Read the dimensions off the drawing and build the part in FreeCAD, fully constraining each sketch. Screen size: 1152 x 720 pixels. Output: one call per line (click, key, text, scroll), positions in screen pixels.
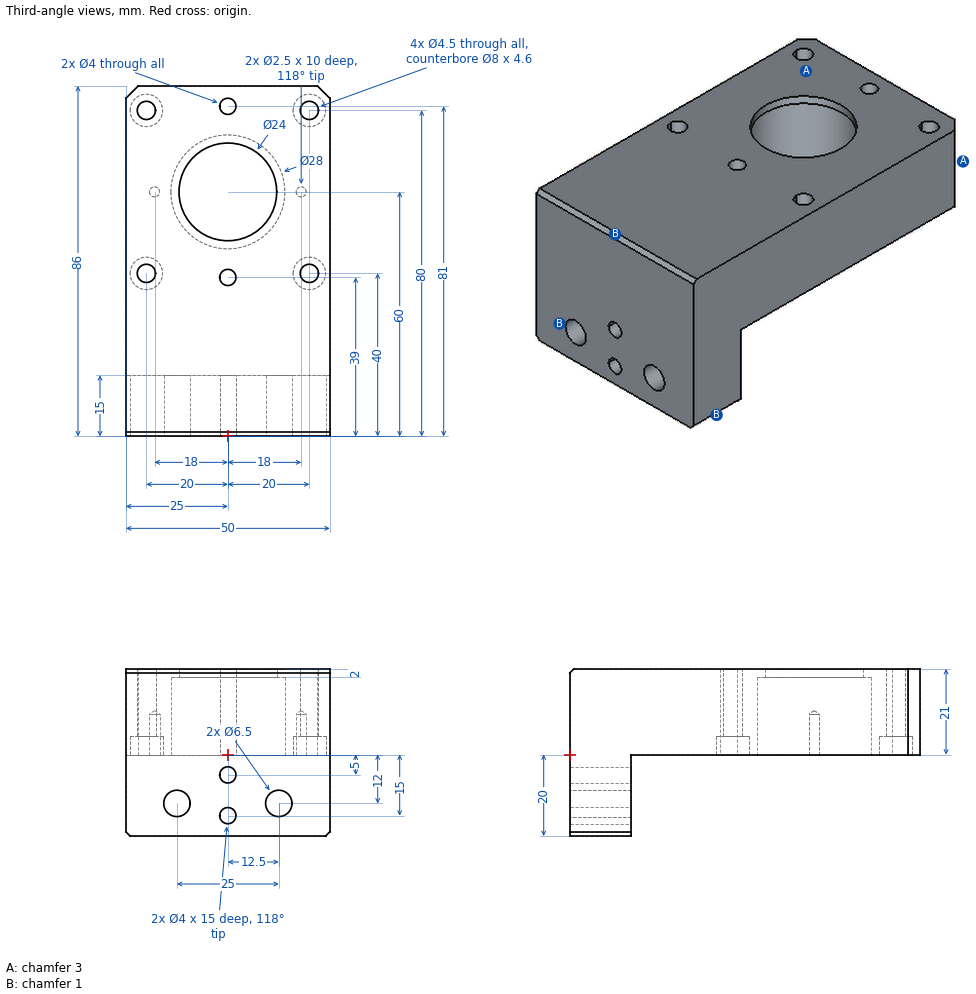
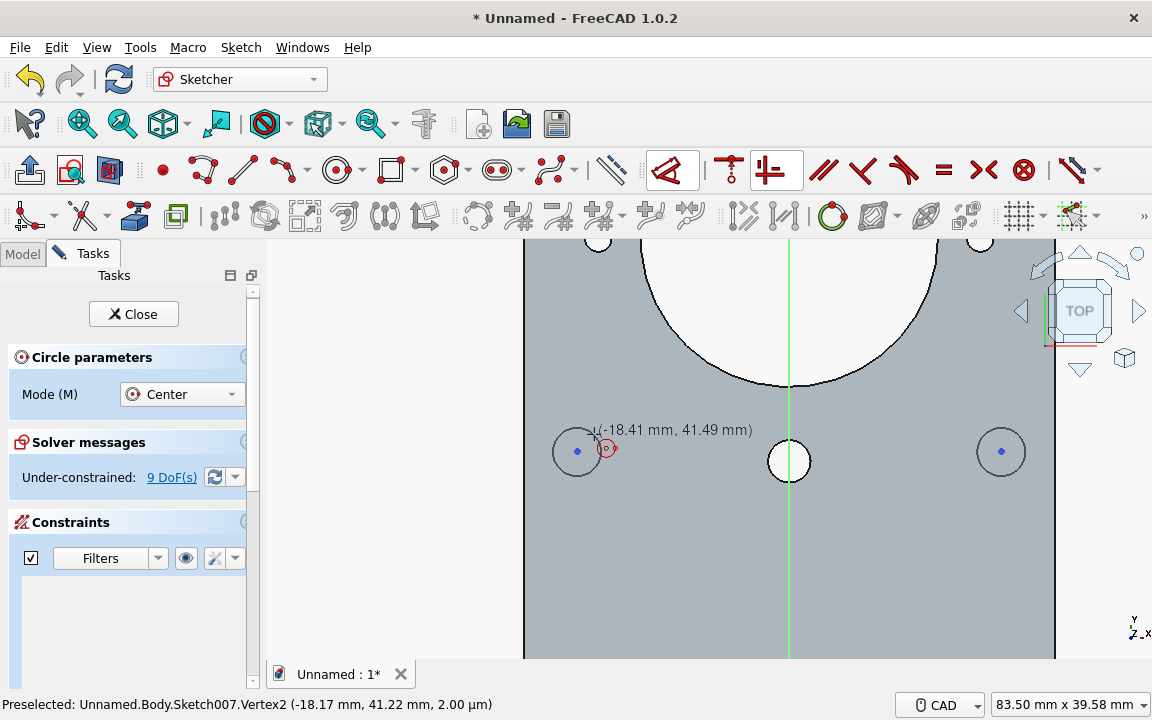
scroll(576, 453, down, 6)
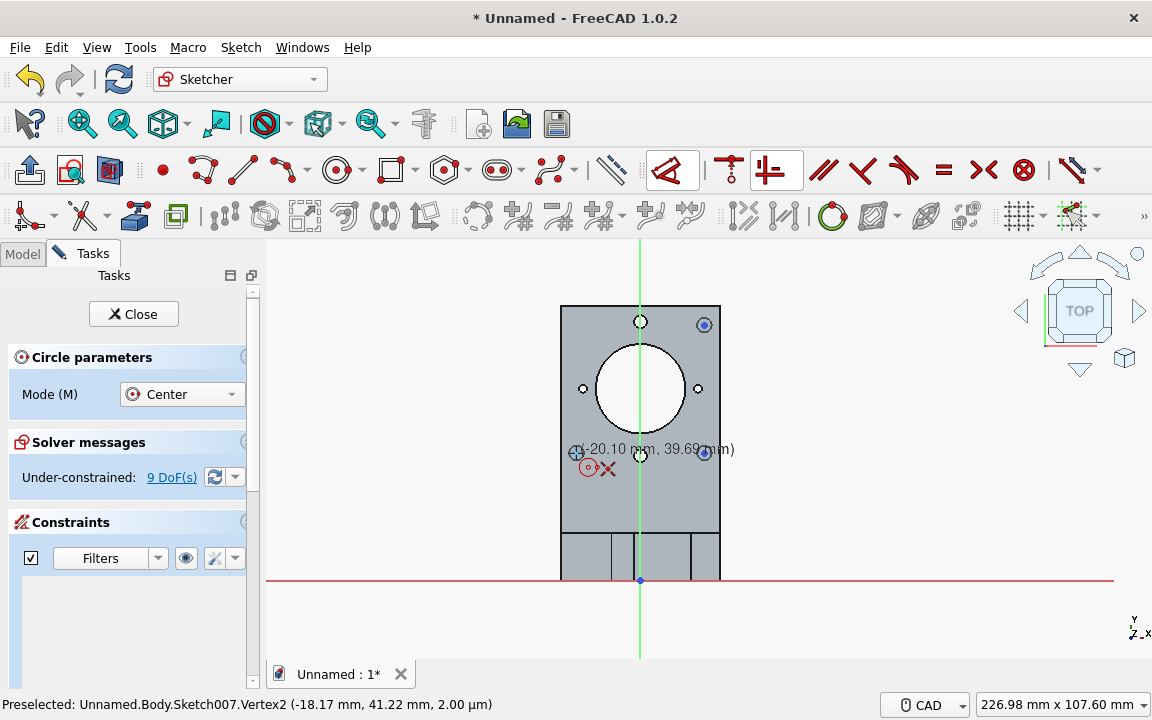
scroll(577, 325, up, 6)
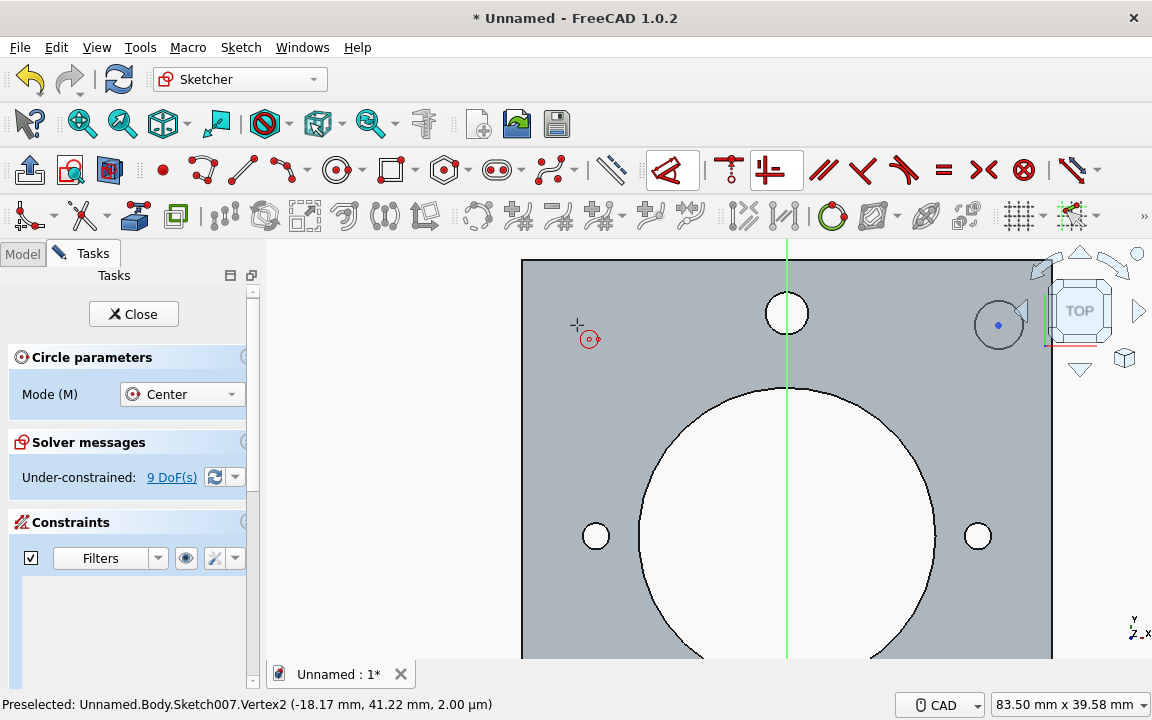
click(575, 324)
click(592, 307)
key(Escape)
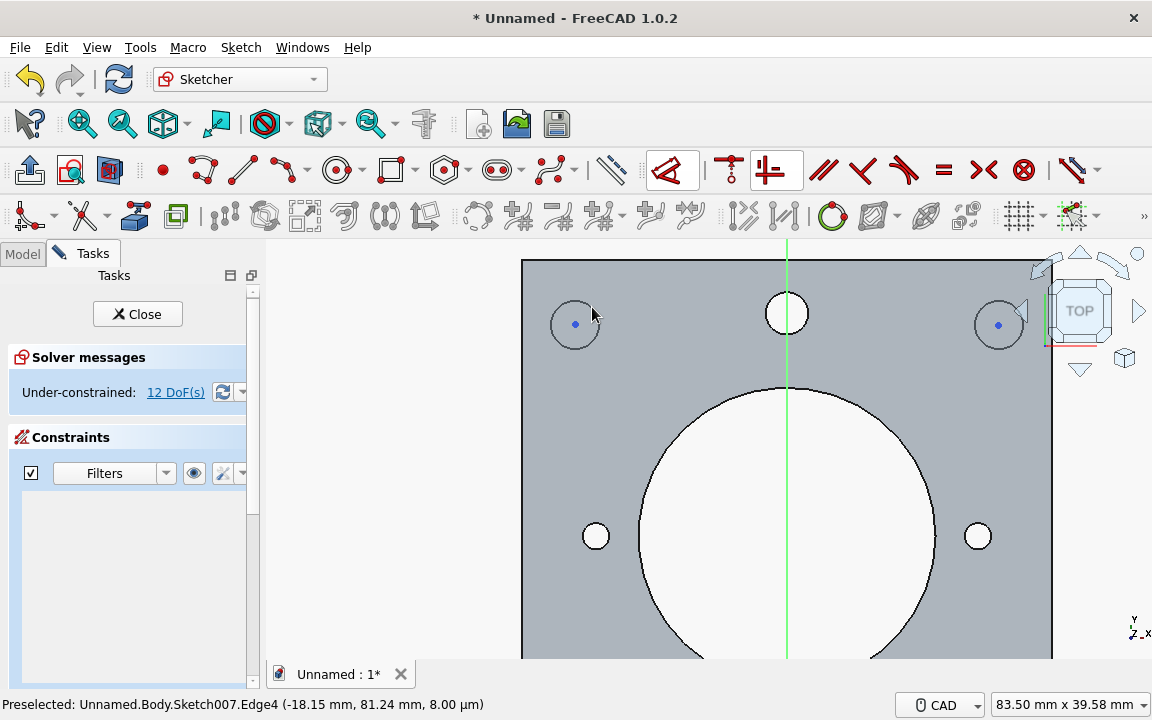
click(982, 308)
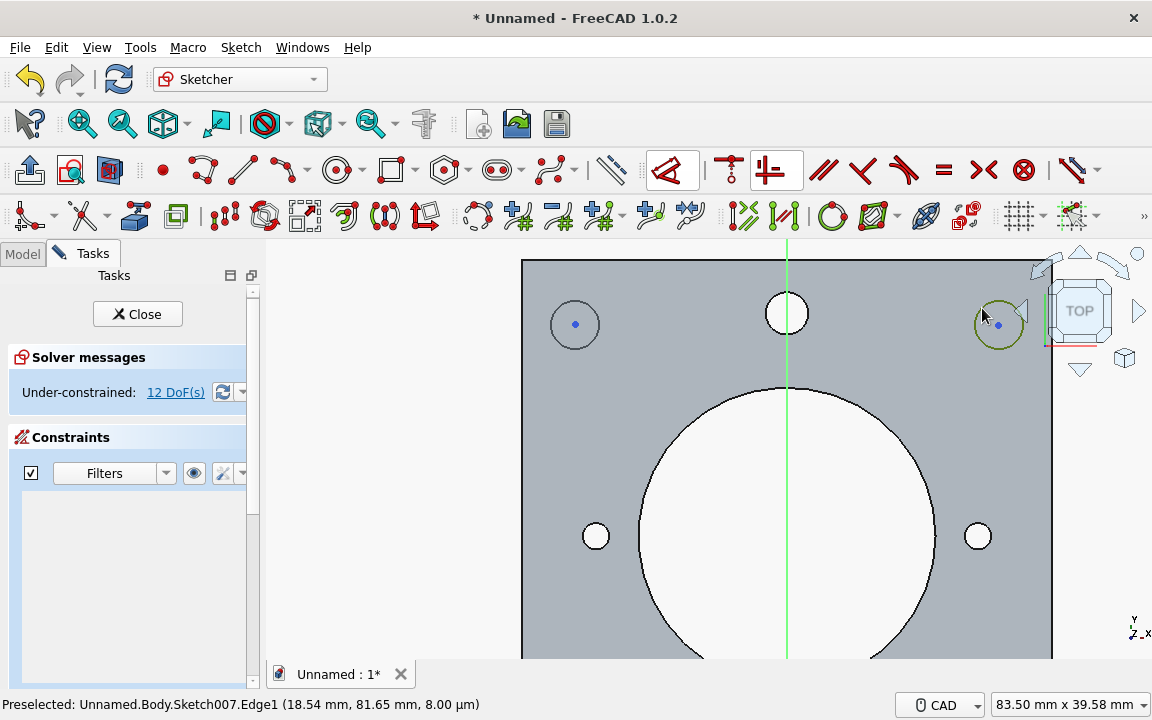
scroll(577, 325, down, 6)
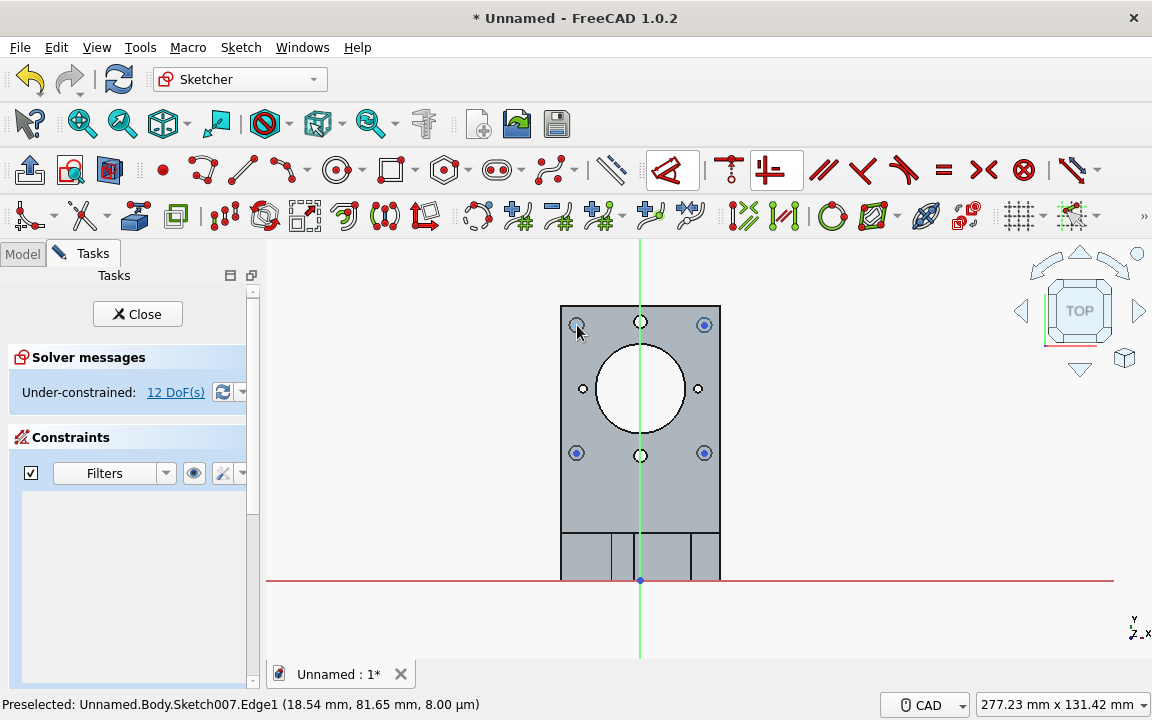
scroll(709, 448, up, 4)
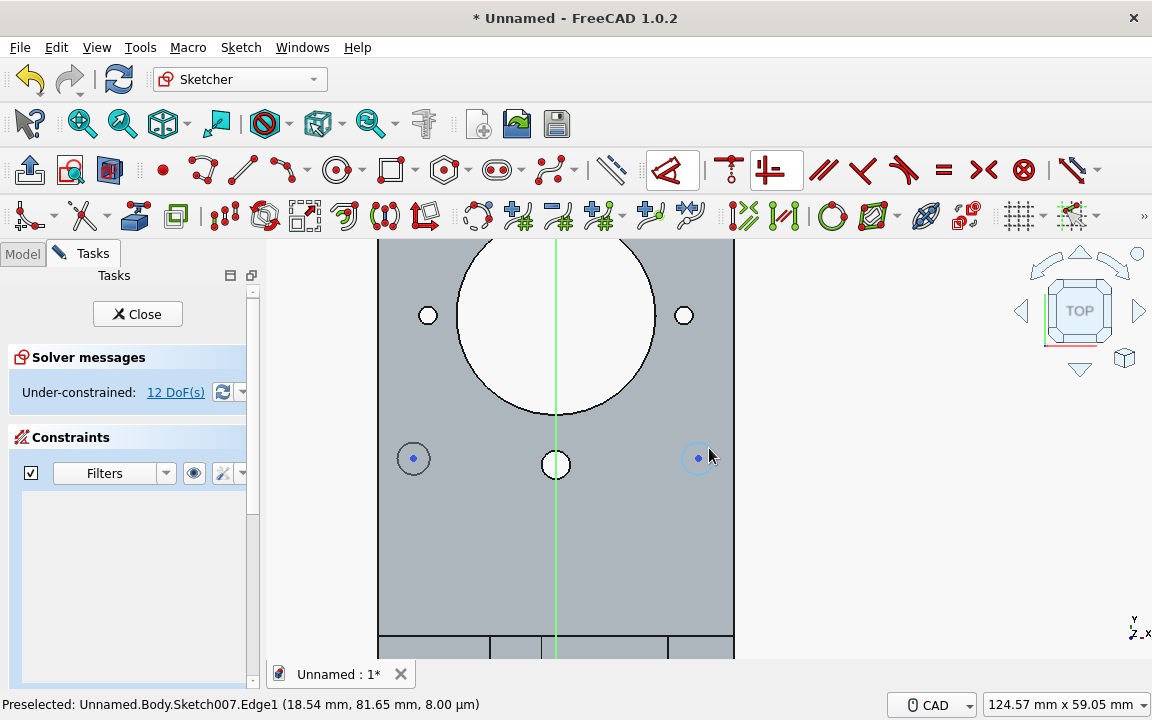
click(709, 447)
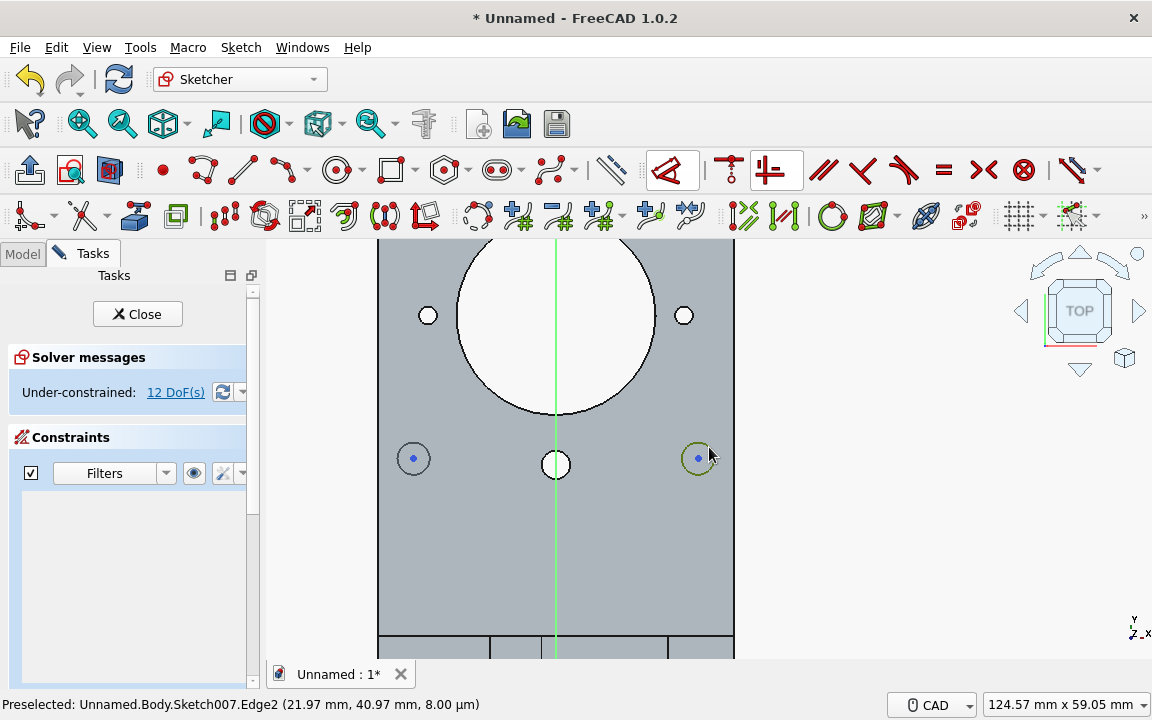
click(425, 447)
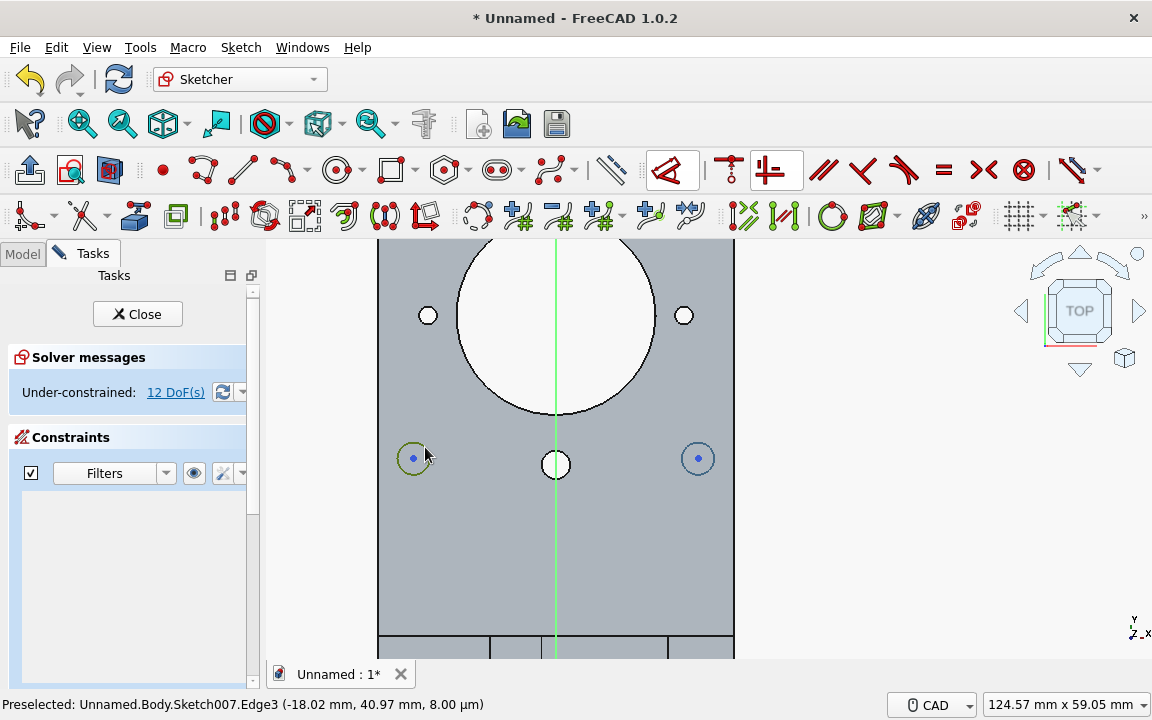
scroll(710, 448, down, 4)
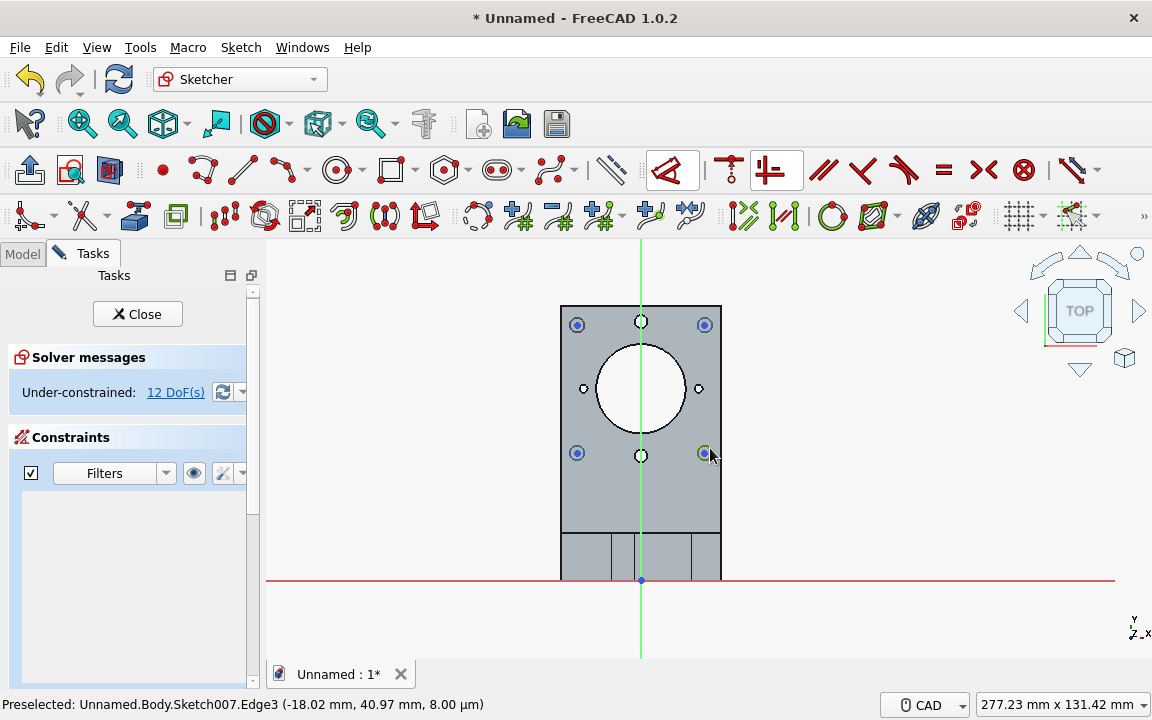
scroll(582, 320, up, 4)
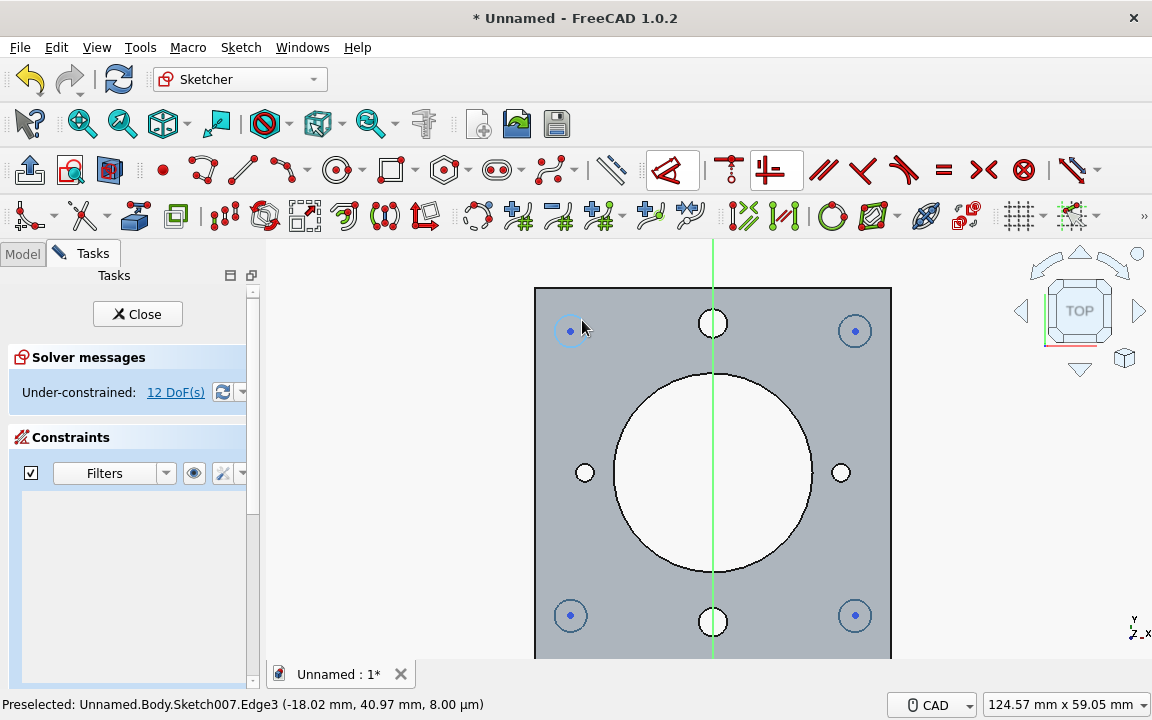
click(582, 320)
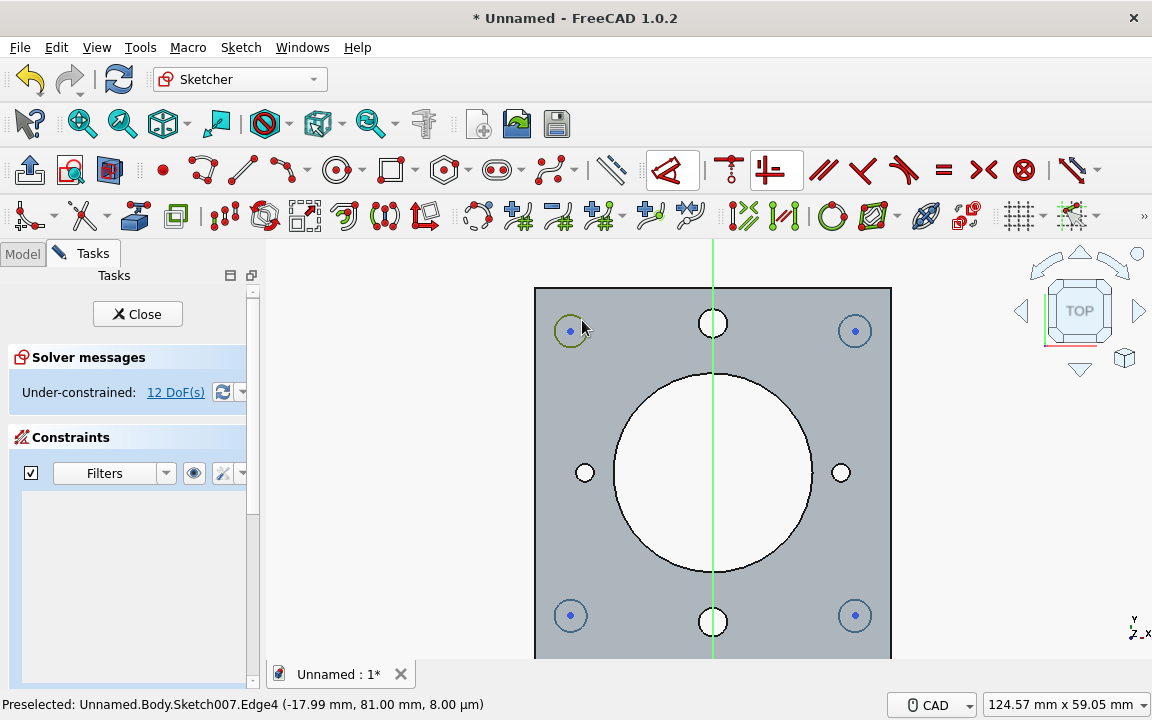
click(944, 170)